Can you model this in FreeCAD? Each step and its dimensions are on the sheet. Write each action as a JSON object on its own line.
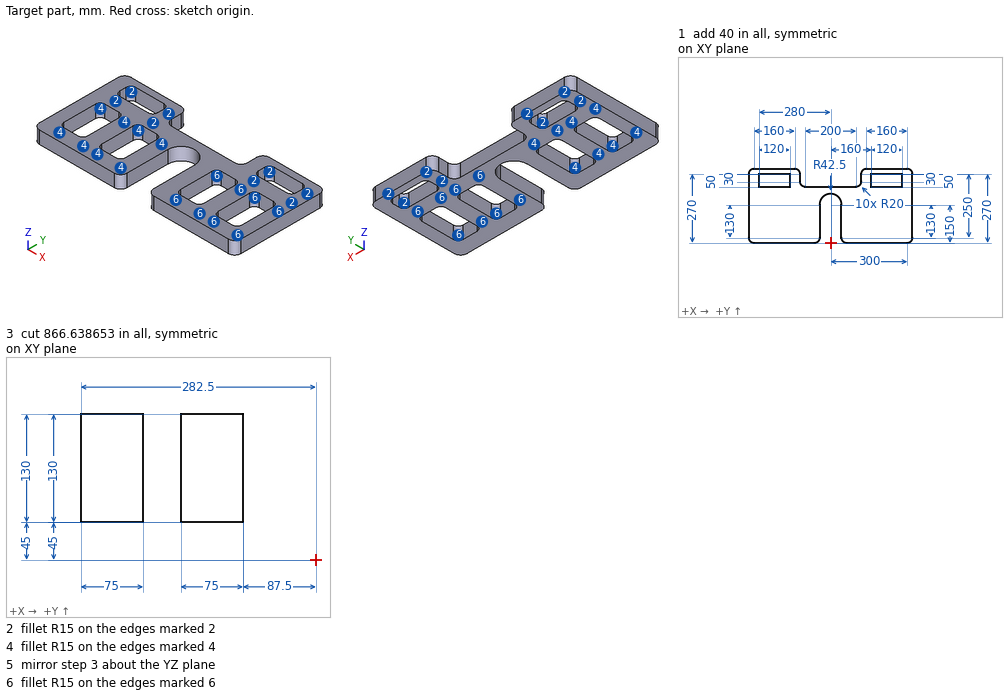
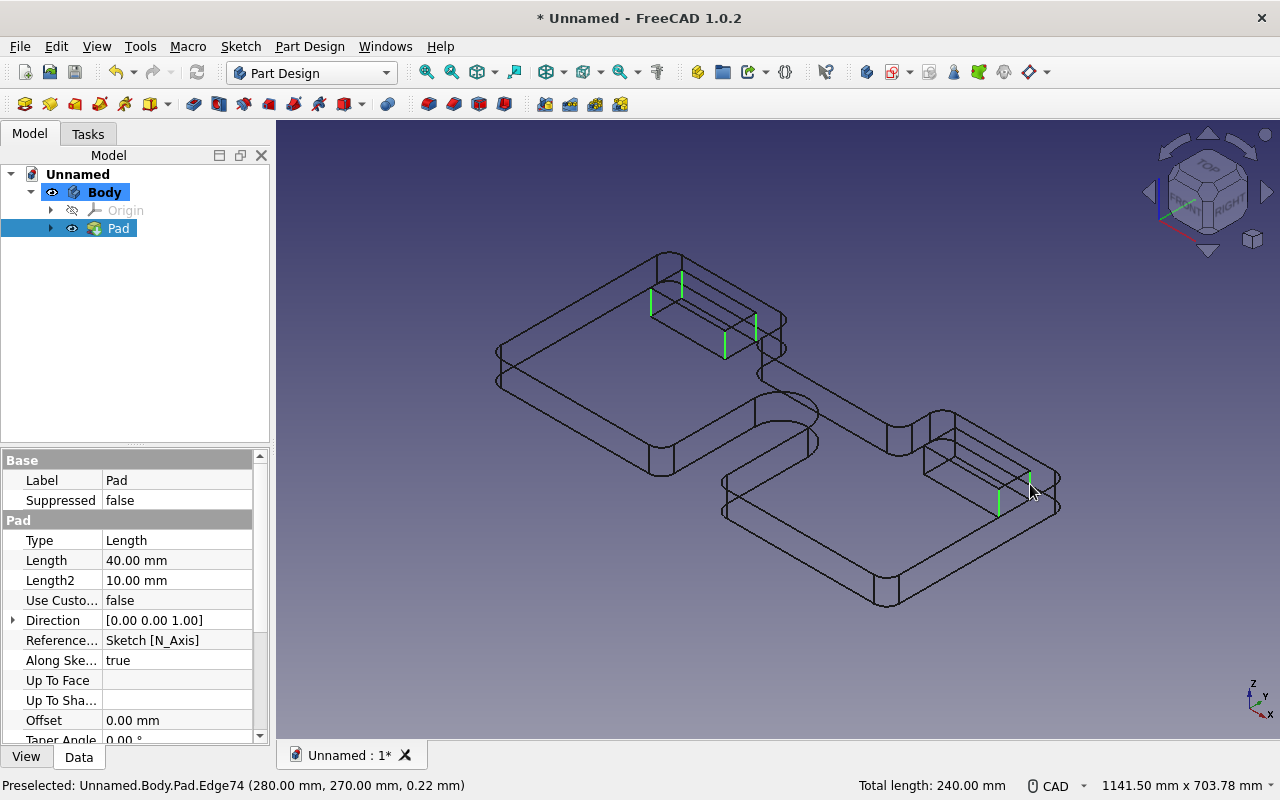
{"action": "left_click", "coordinate": [955, 441], "text": "ctrl"}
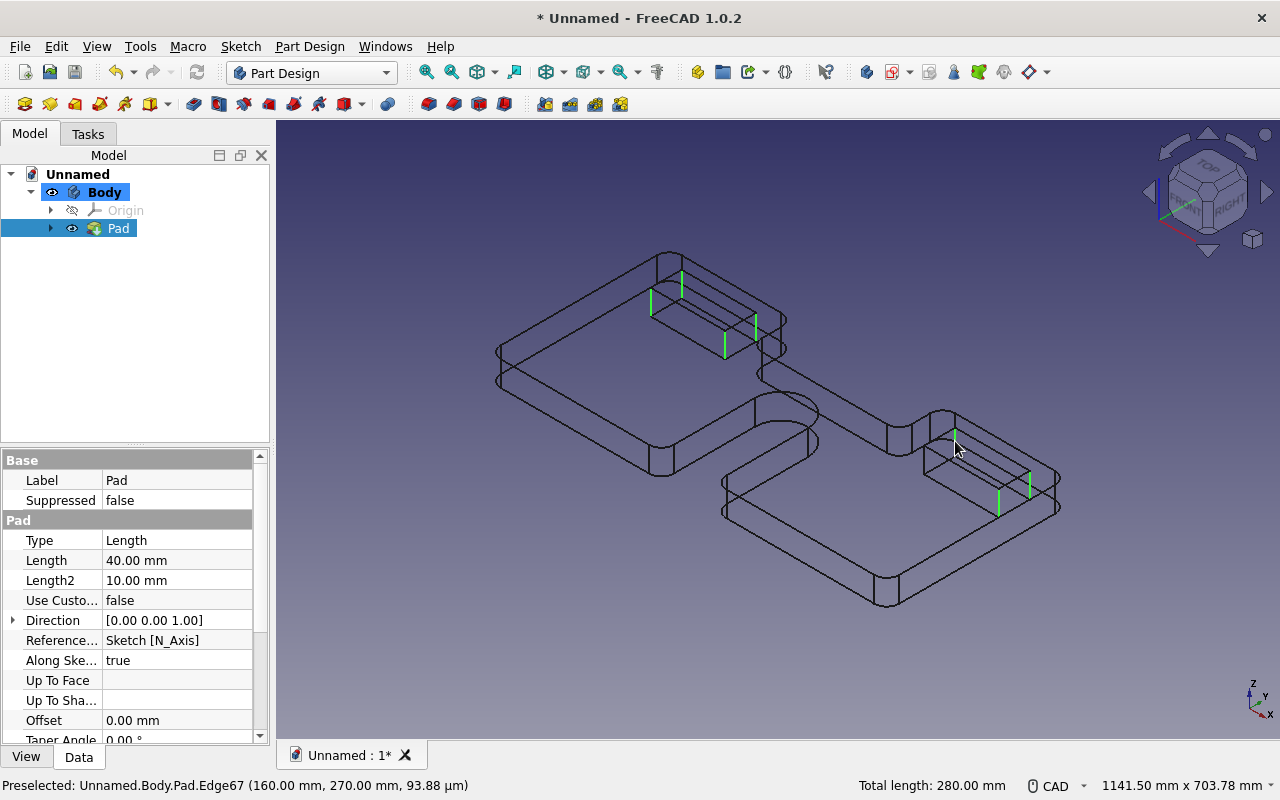
{"action": "left_click", "coordinate": [924, 459], "text": "ctrl"}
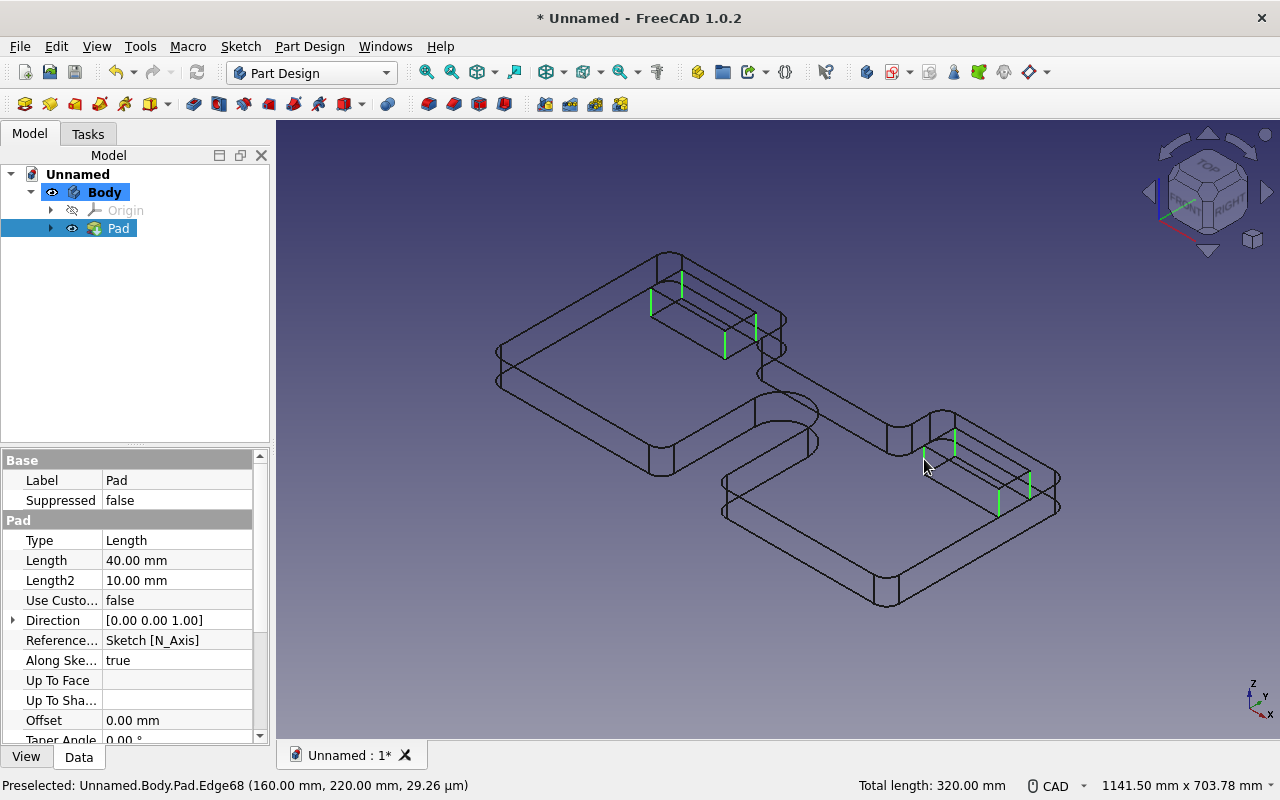
{"action": "key", "text": "v 1"}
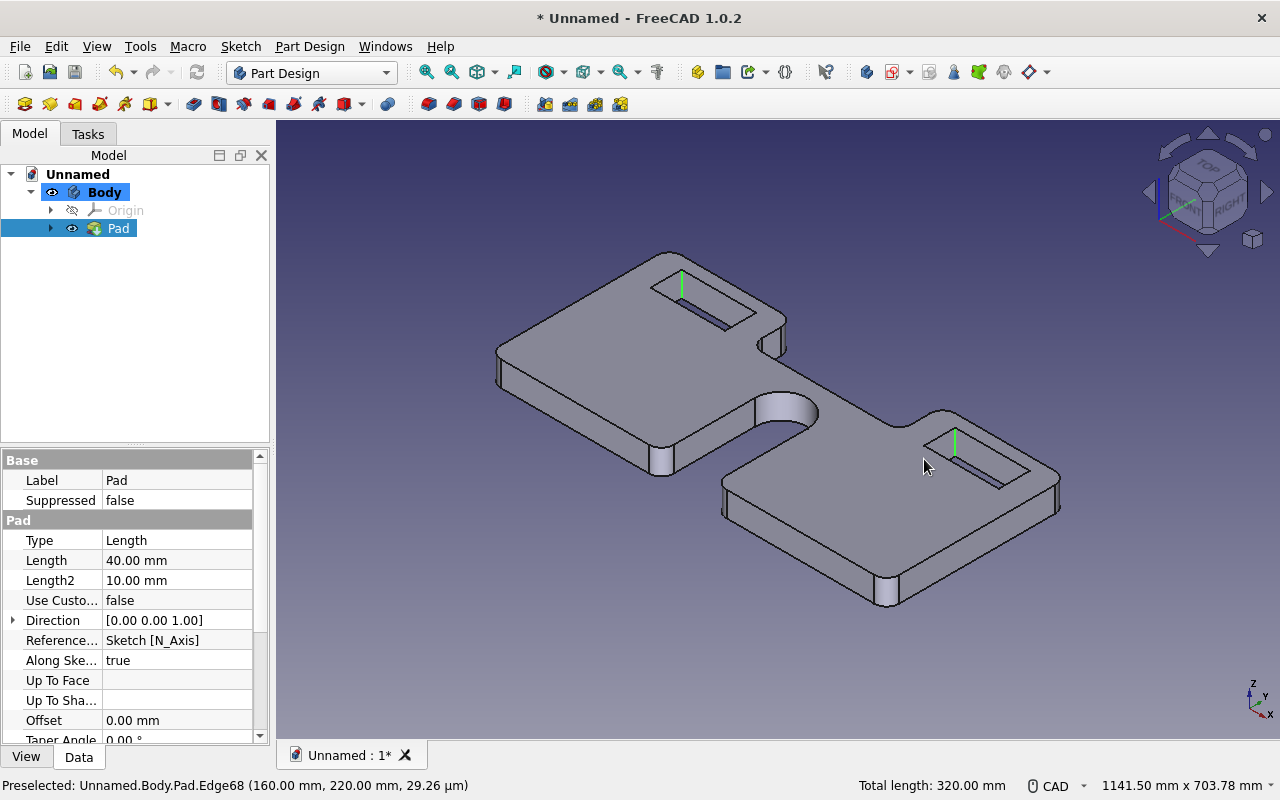
{"action": "left_click", "coordinate": [429, 104]}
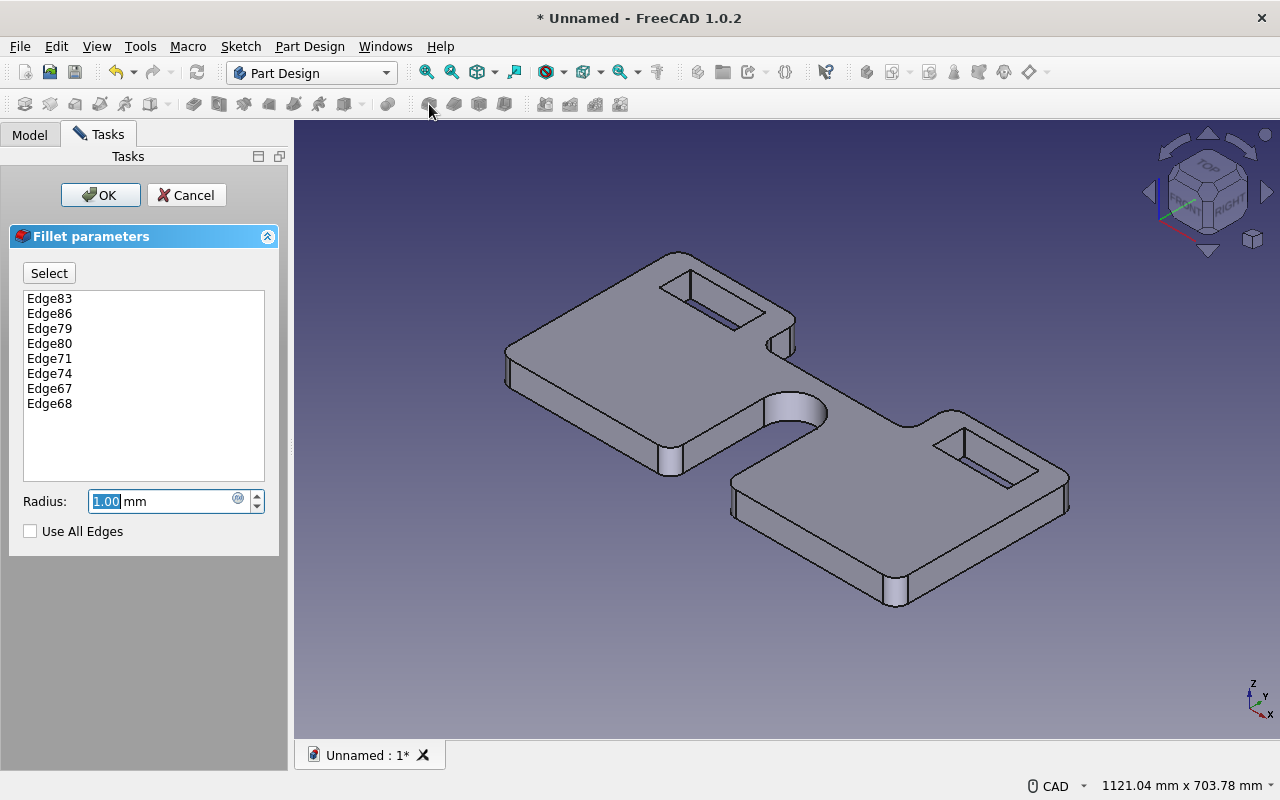
{"action": "type", "text": "15"}
{"action": "key", "text": "Tab"}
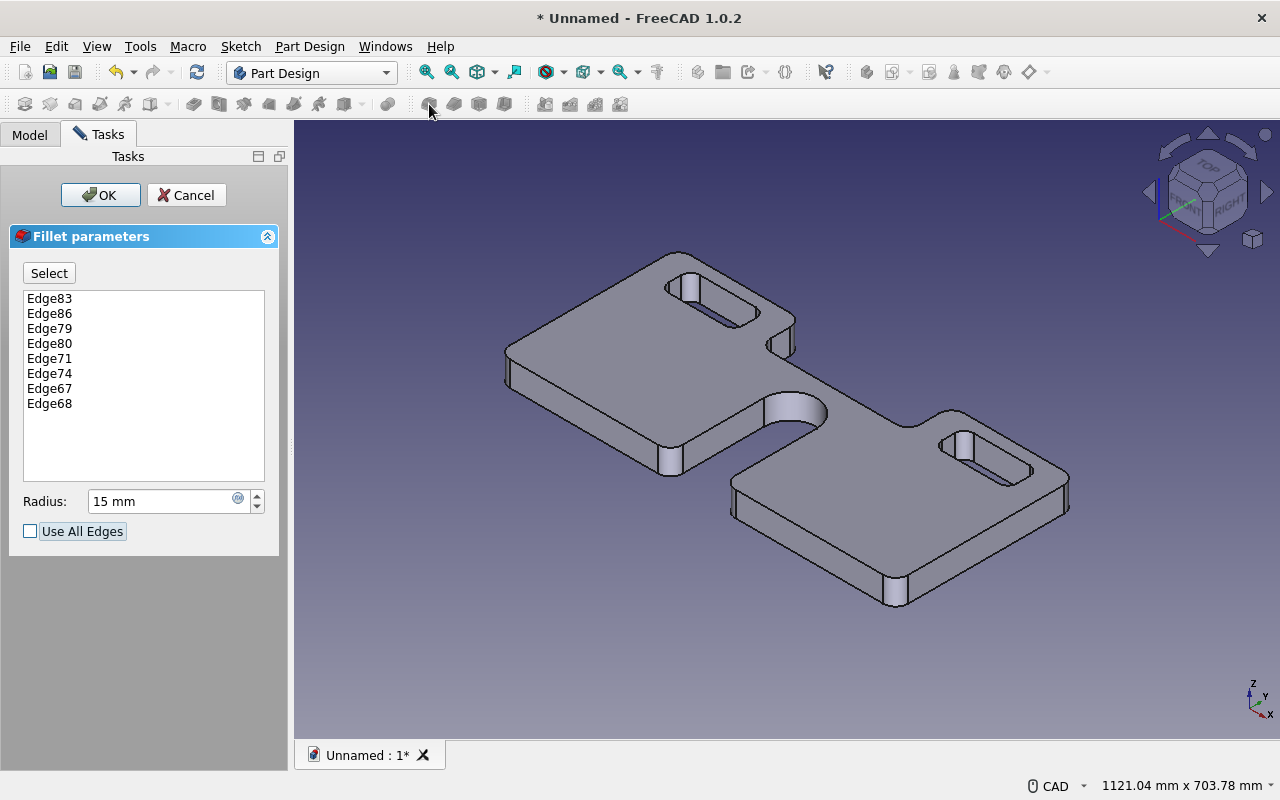
{"action": "left_click", "coordinate": [101, 195]}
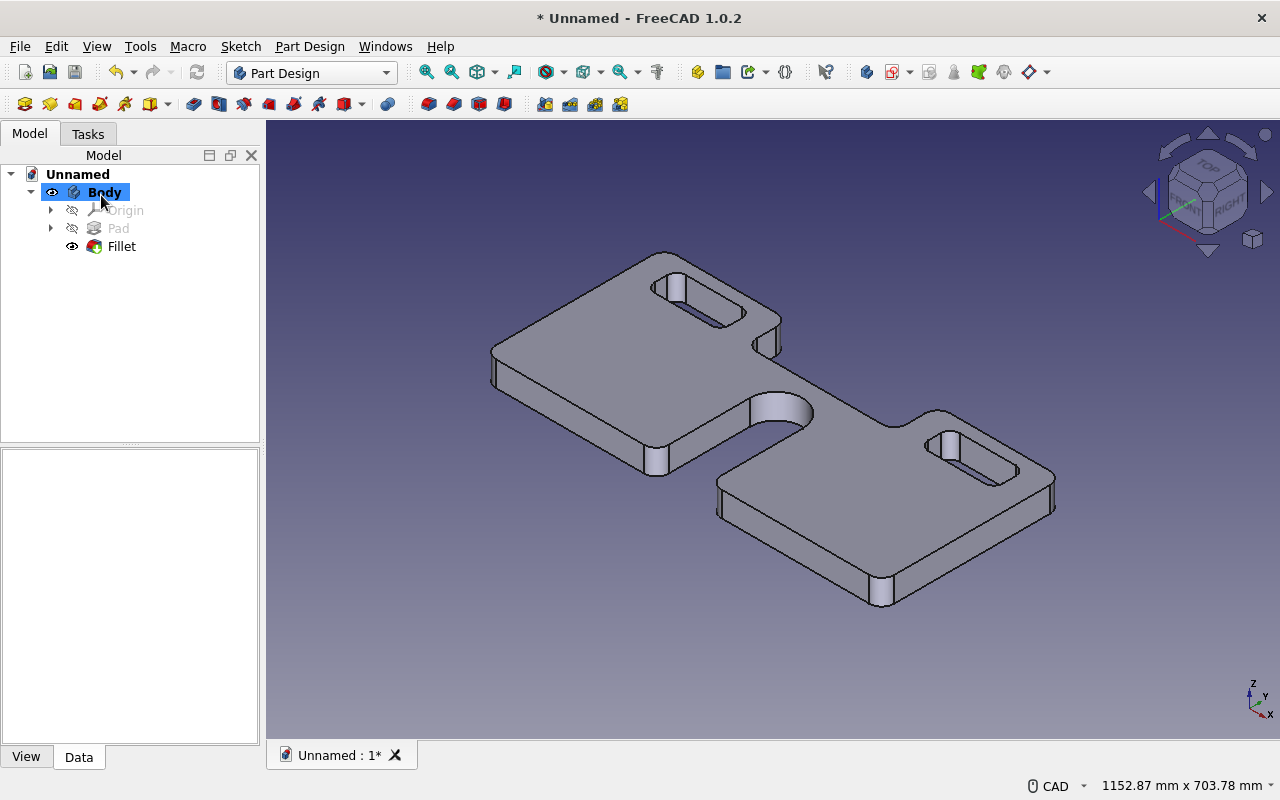
{"action": "left_click", "coordinate": [892, 72]}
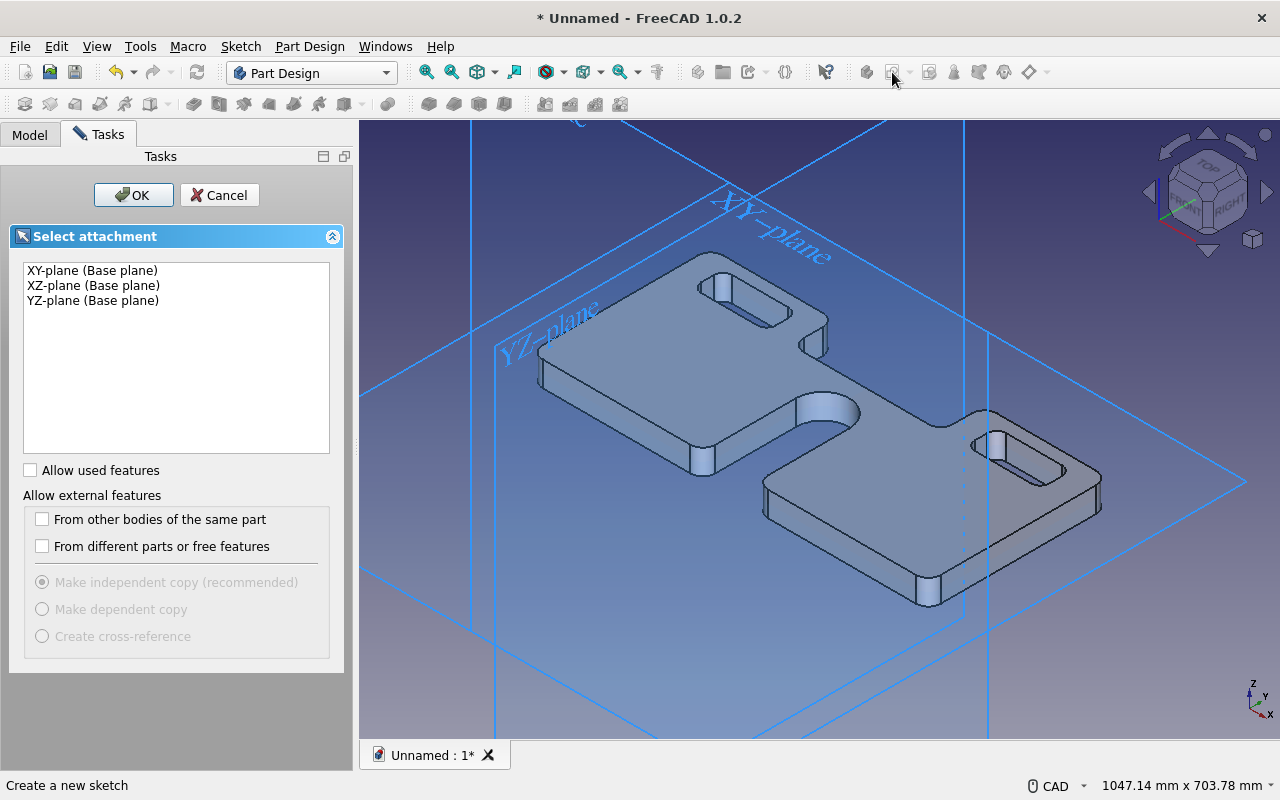
{"action": "left_click", "coordinate": [84, 270]}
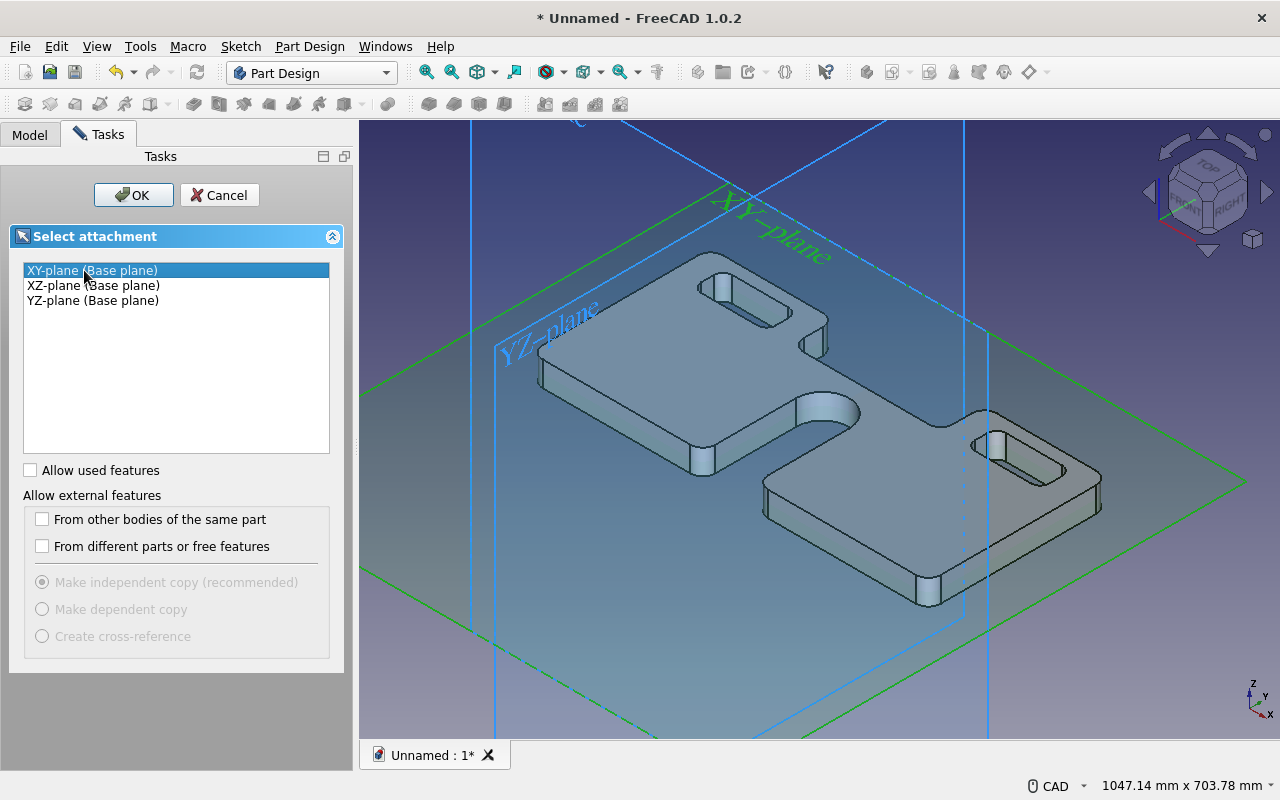
{"action": "left_click", "coordinate": [134, 195]}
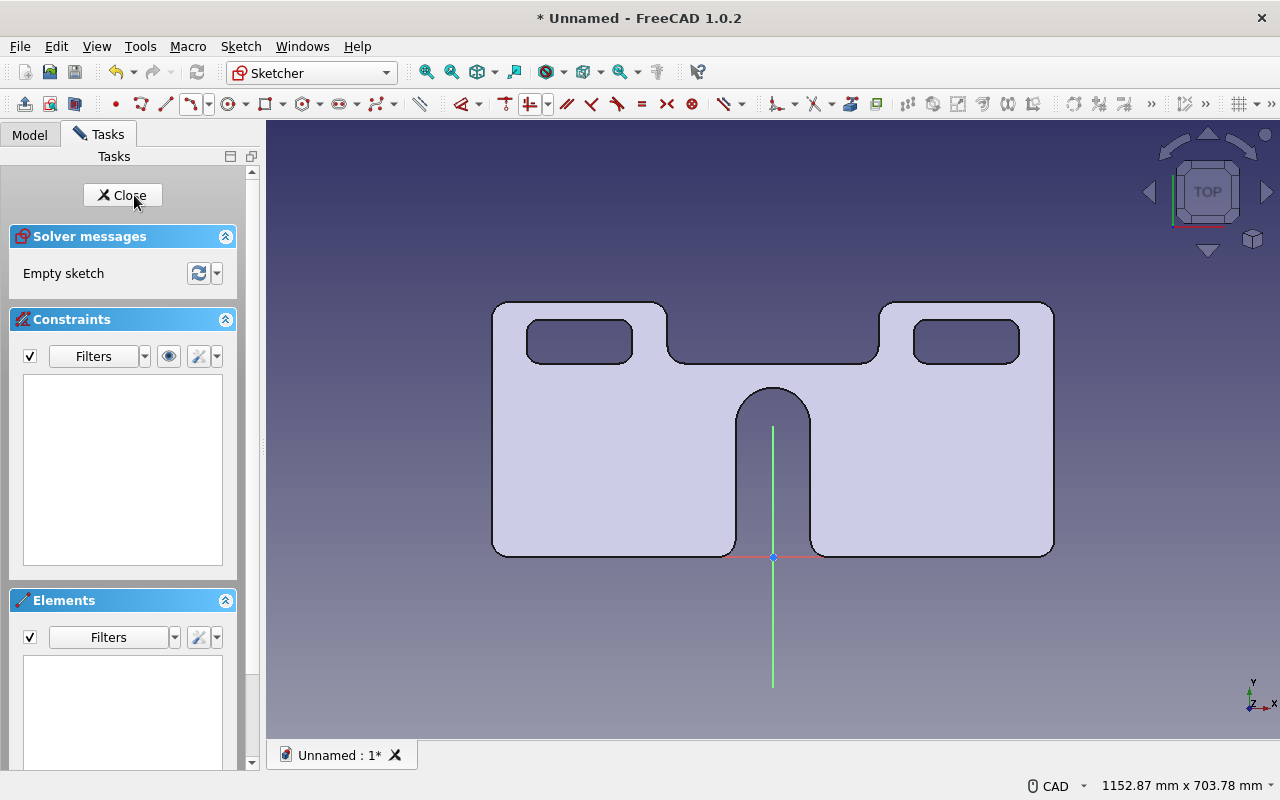
{"action": "key", "text": "q s"}